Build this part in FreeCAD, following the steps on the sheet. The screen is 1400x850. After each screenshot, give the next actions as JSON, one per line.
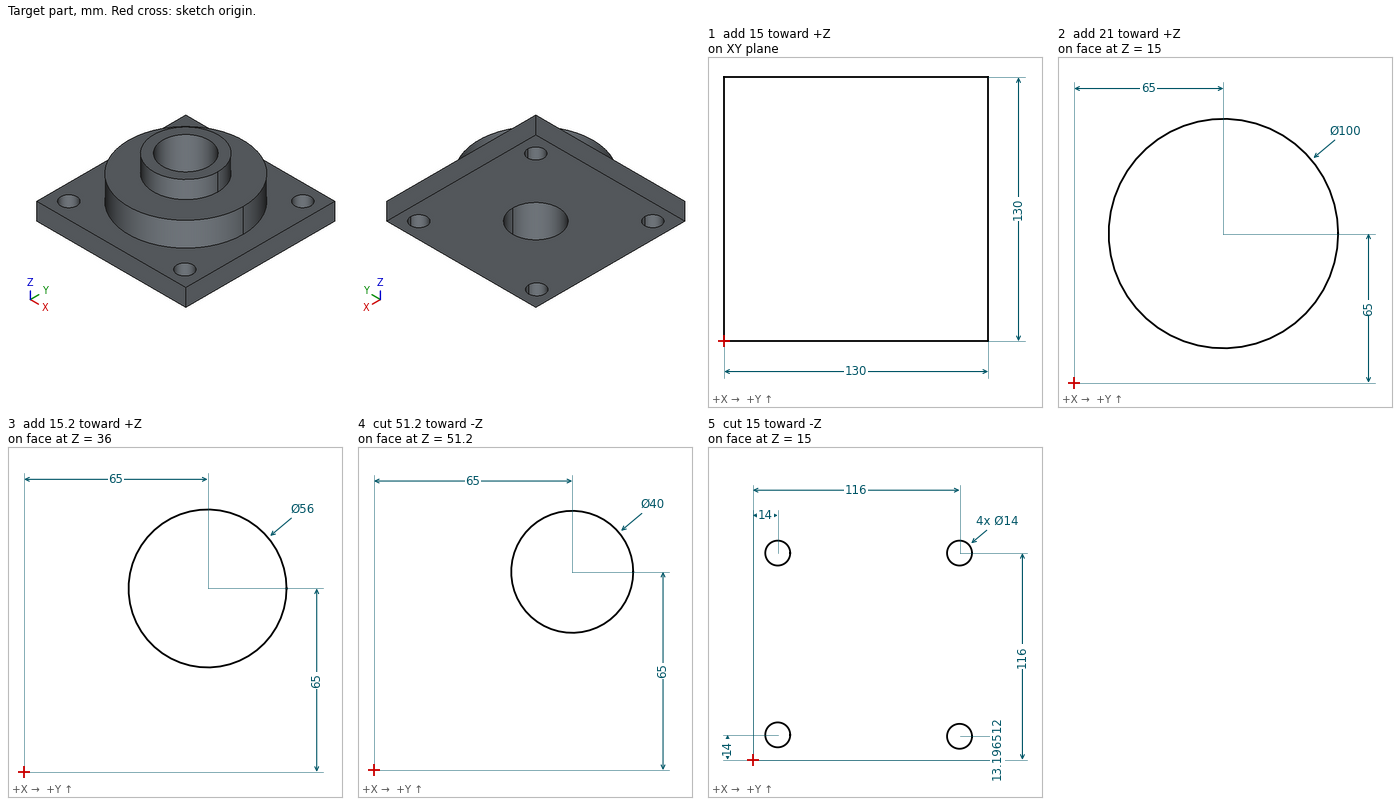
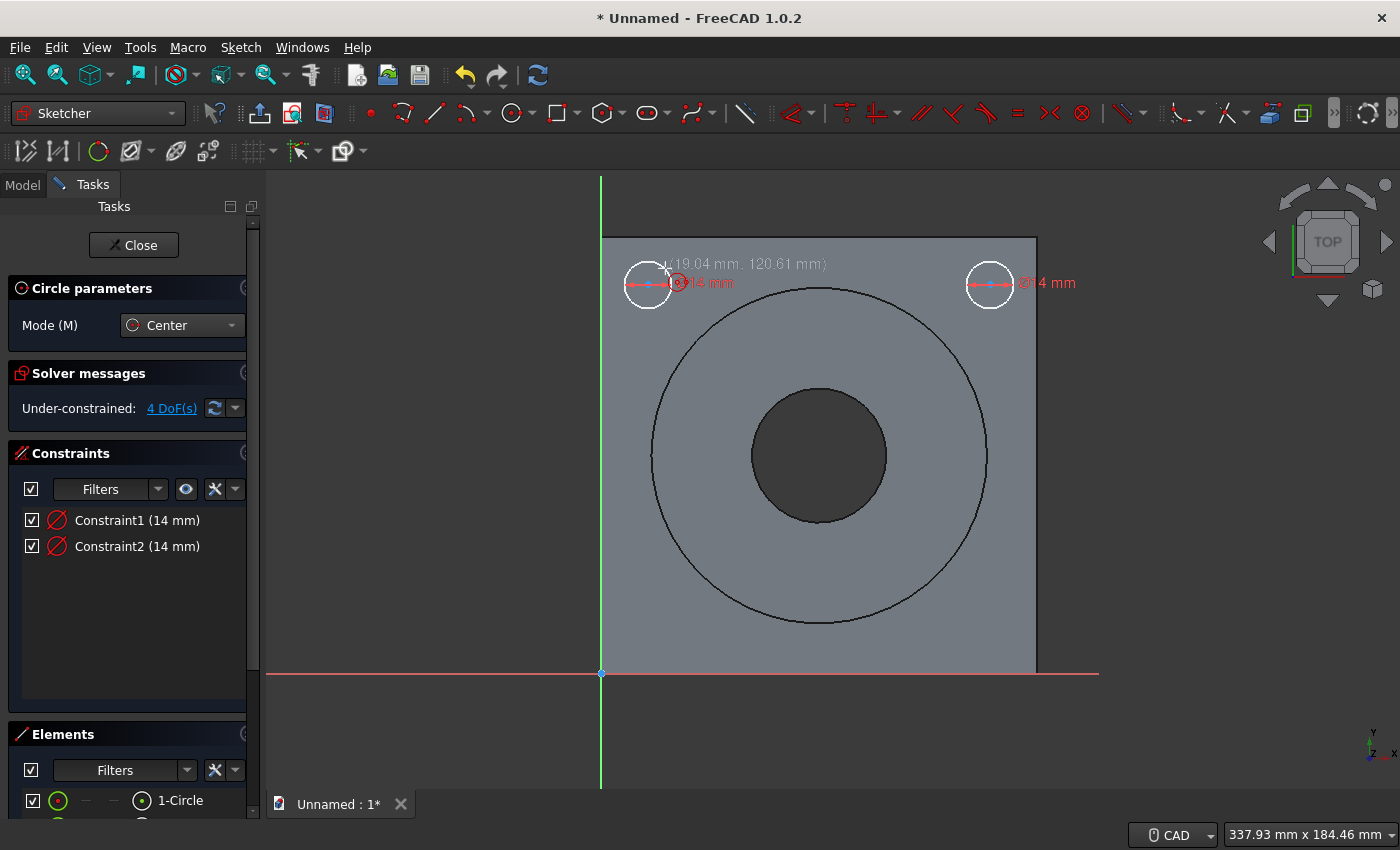
{"action": "left_click", "coordinate": [648, 627]}
{"action": "mouse_move", "coordinate": [665, 610]}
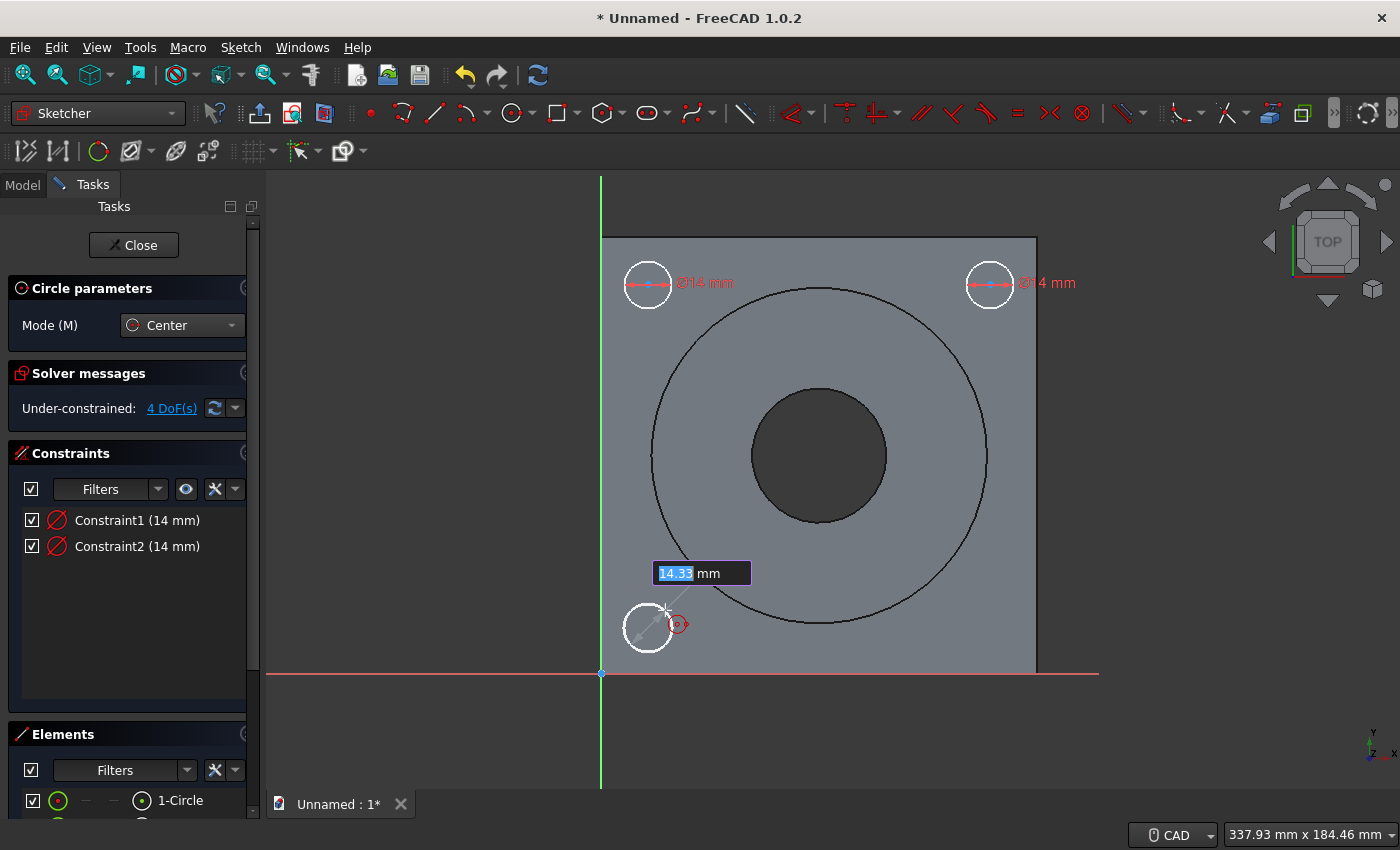
{"action": "type", "text": "14"}
{"action": "key", "text": "Return"}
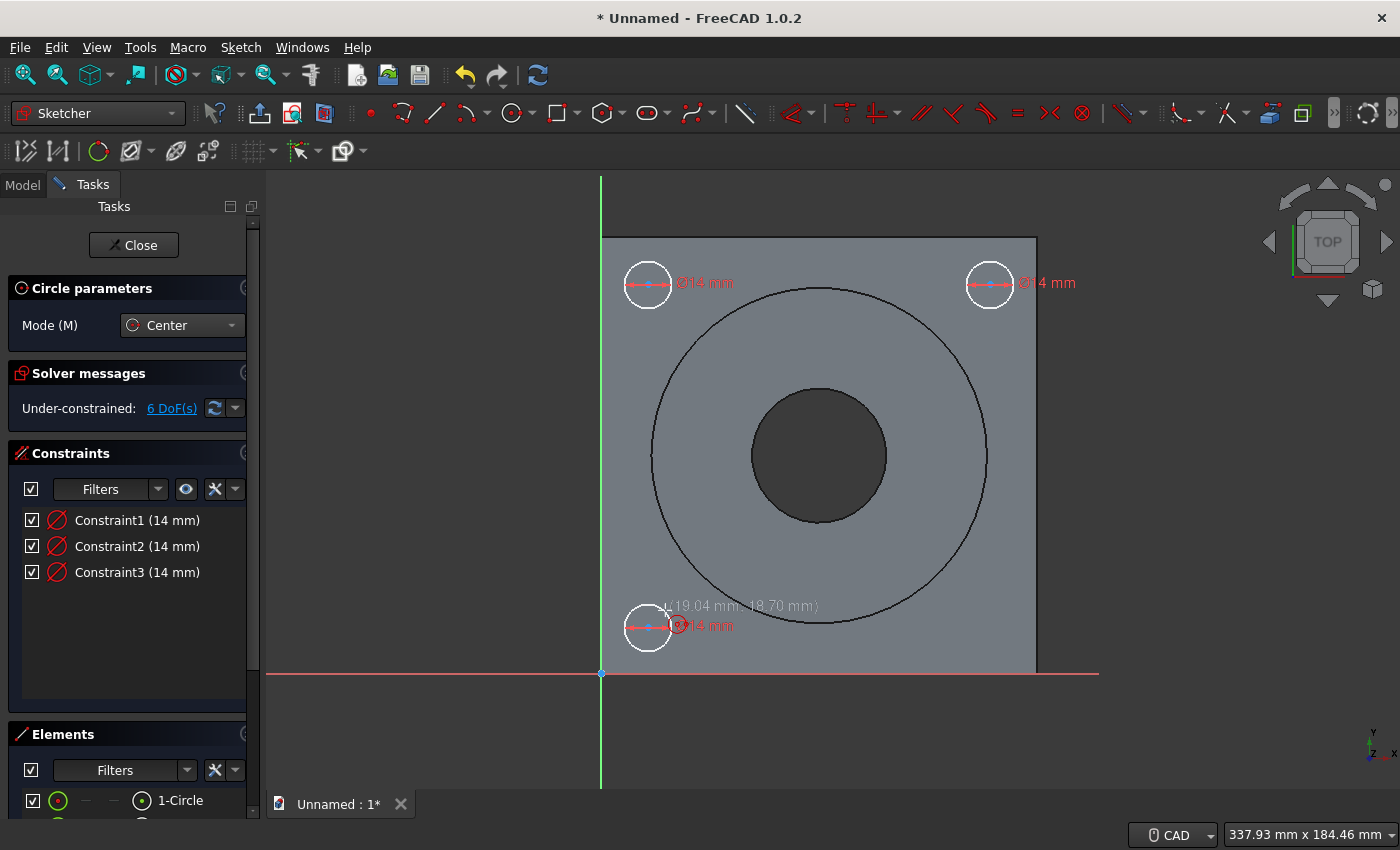
{"action": "left_click", "coordinate": [990, 629]}
{"action": "mouse_move", "coordinate": [1007, 613]}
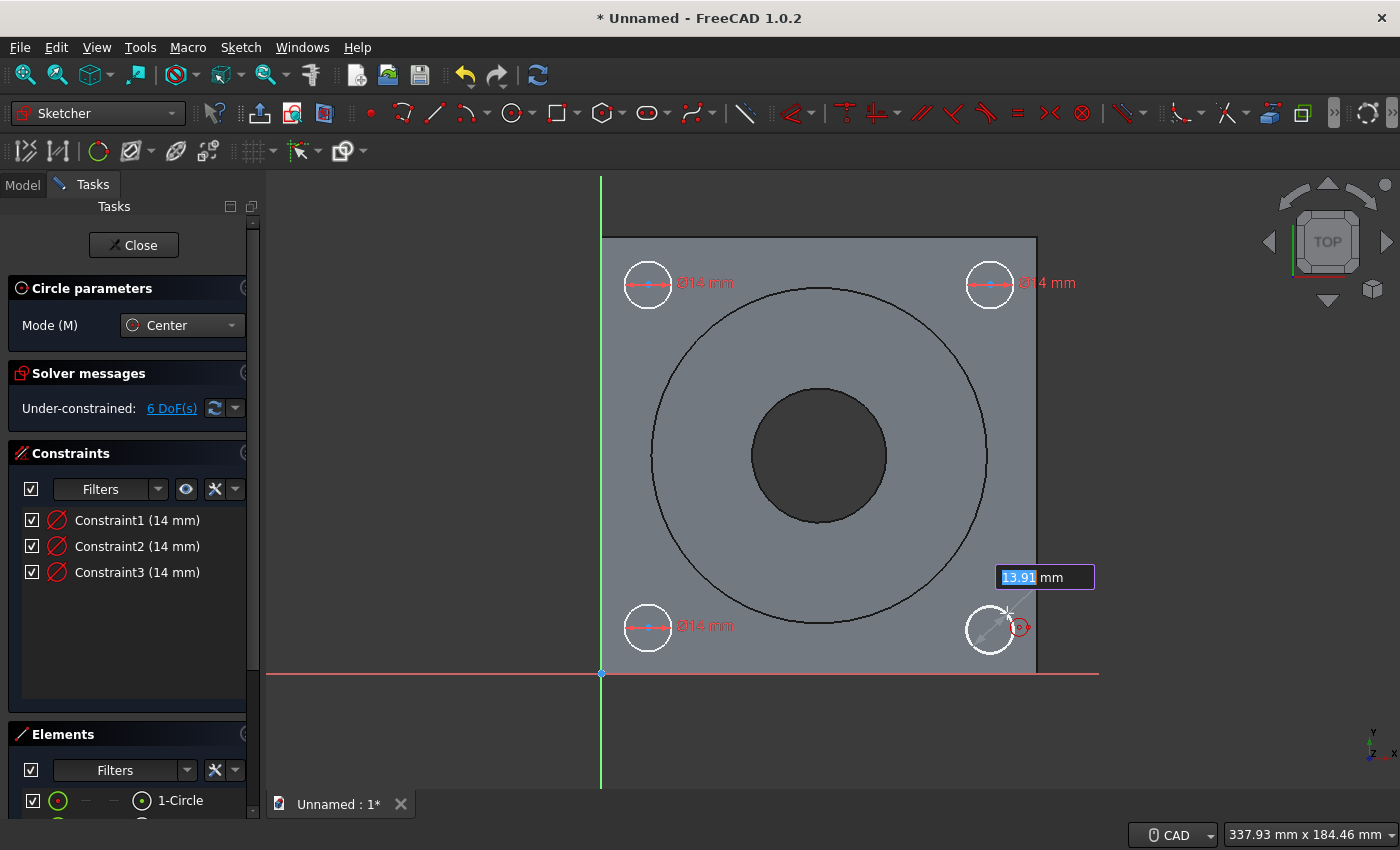
{"action": "type", "text": "14"}
{"action": "key", "text": "Return"}
{"action": "key", "text": "Escape"}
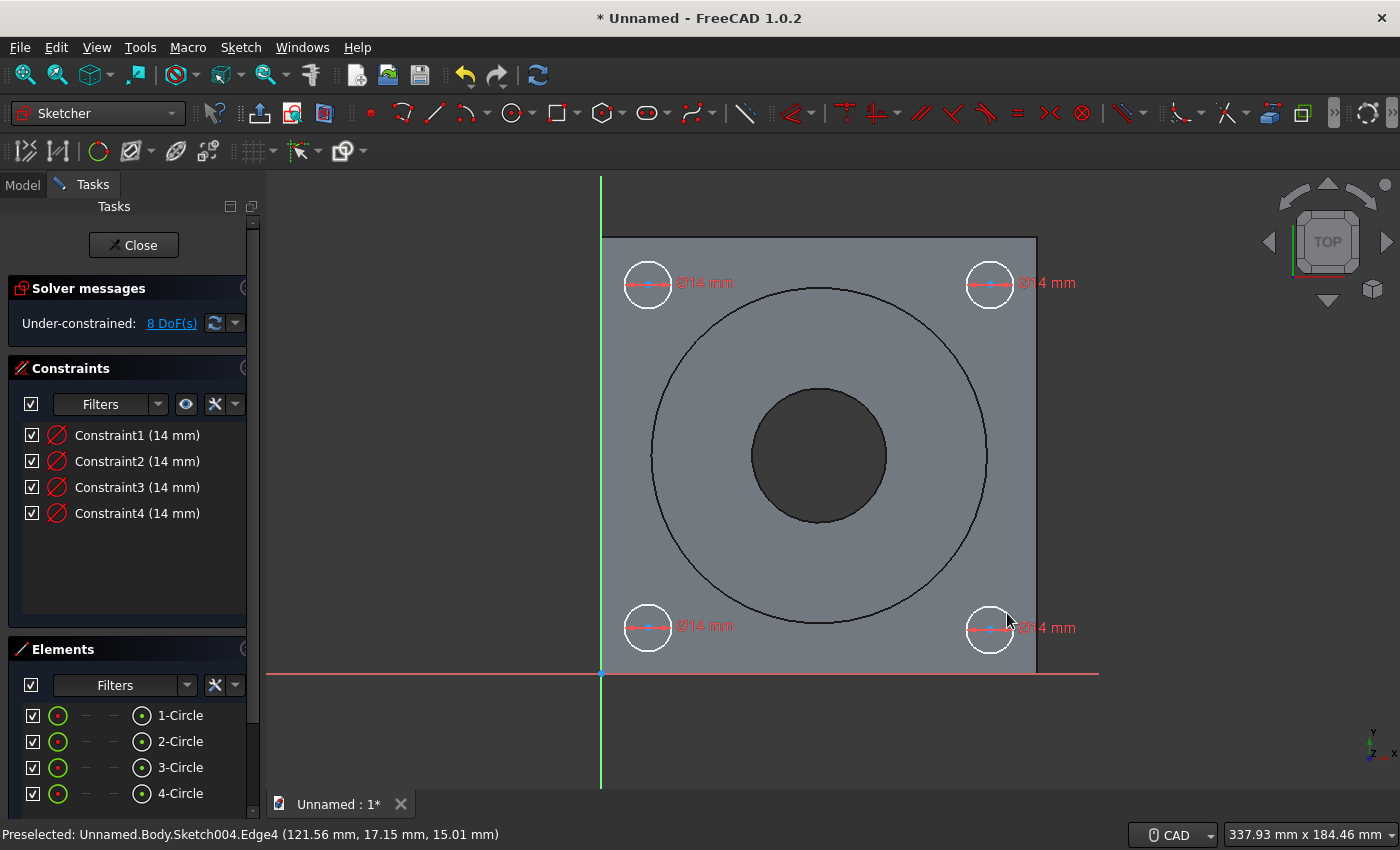
{"action": "left_click", "coordinate": [990, 285]}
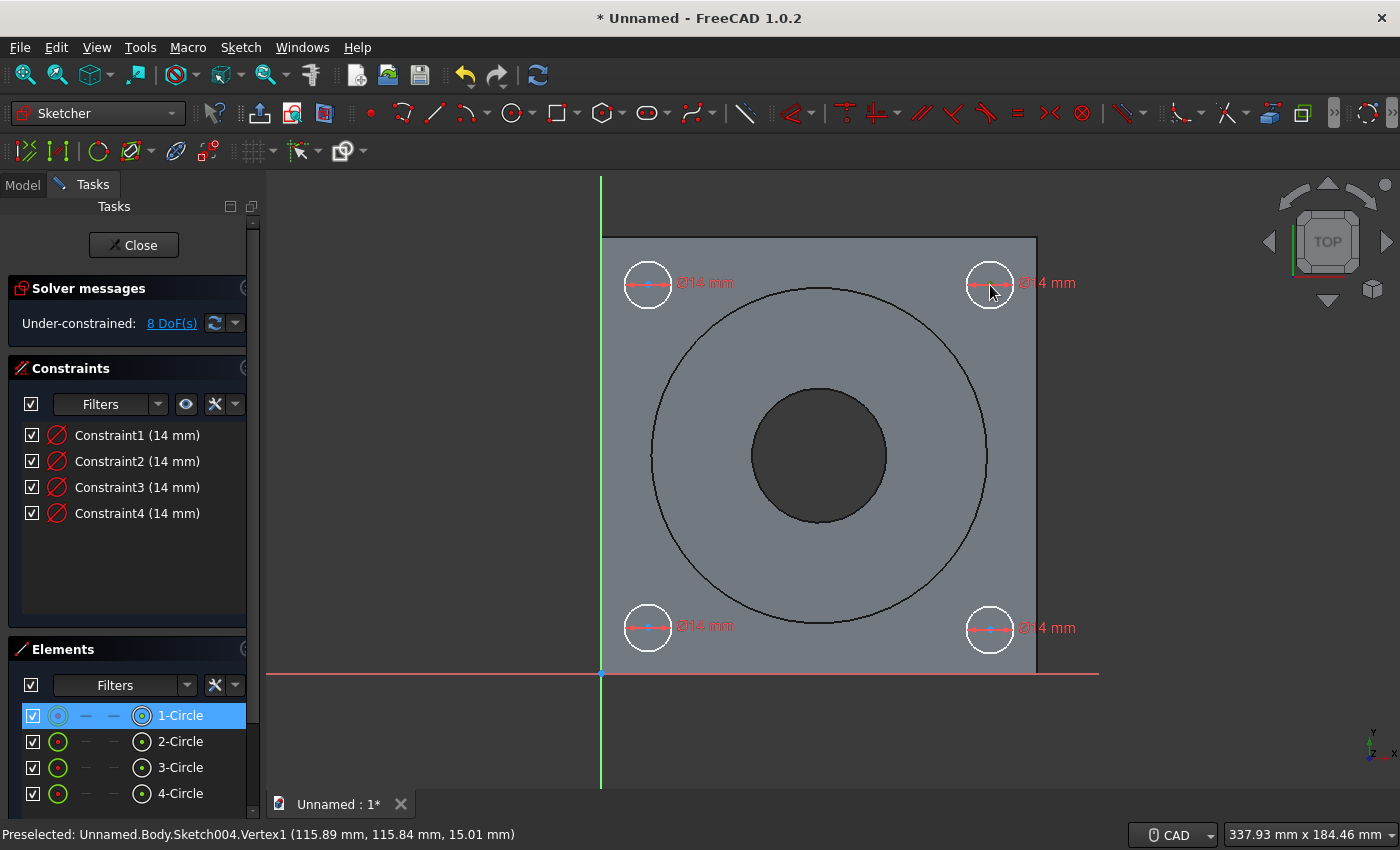
{"action": "left_click", "coordinate": [648, 285]}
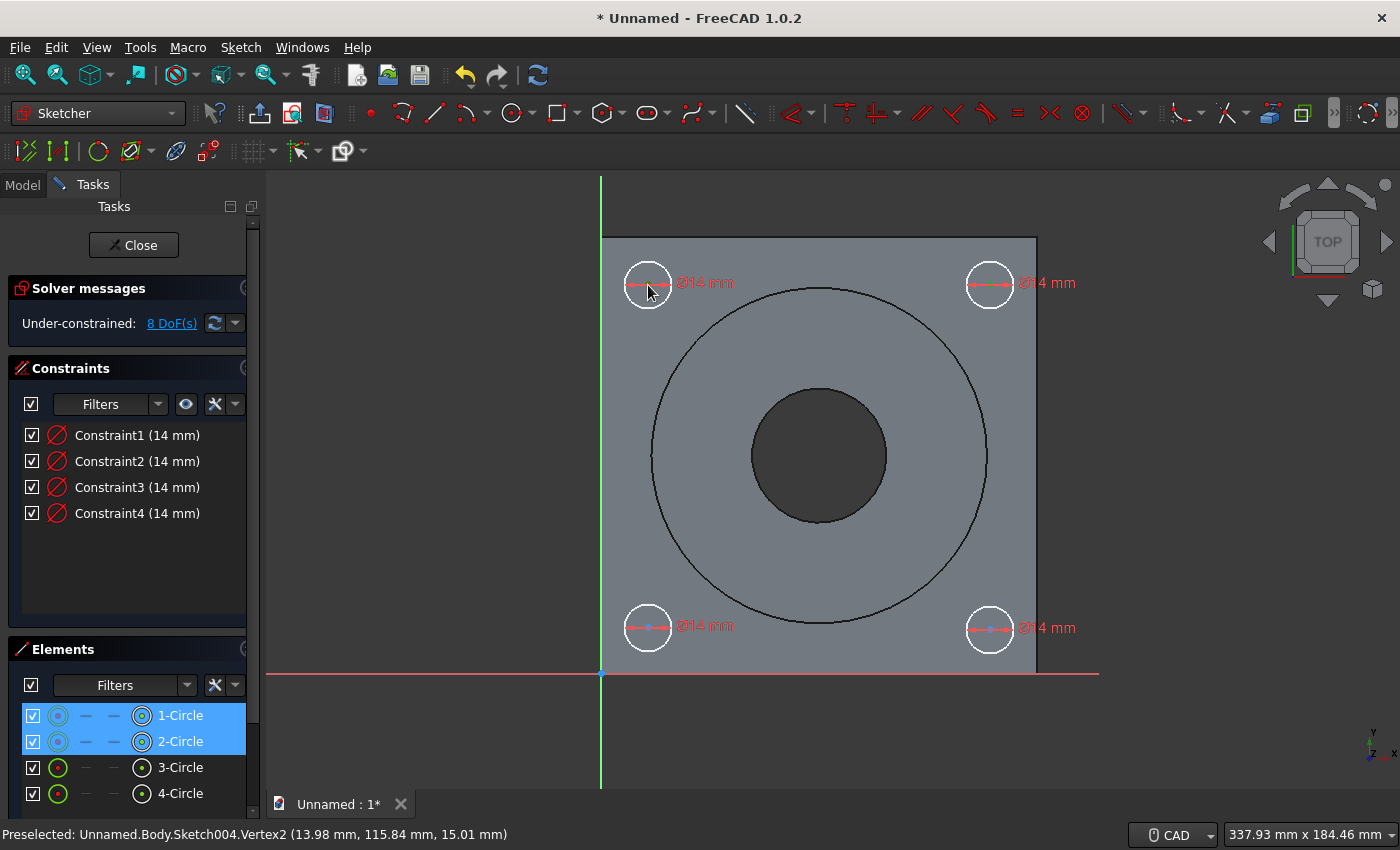
{"action": "key", "text": "h"}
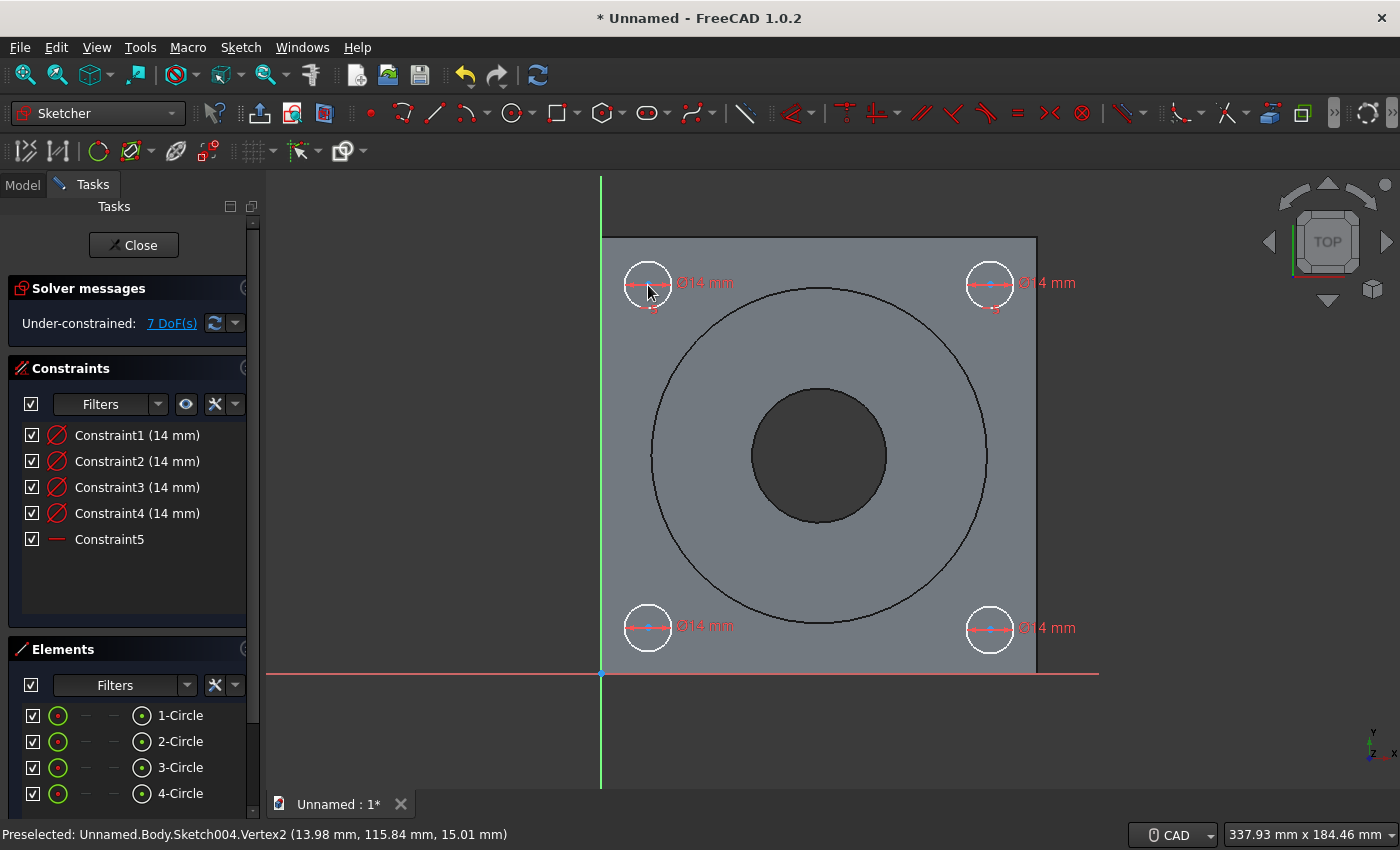
{"action": "left_click", "coordinate": [648, 285]}